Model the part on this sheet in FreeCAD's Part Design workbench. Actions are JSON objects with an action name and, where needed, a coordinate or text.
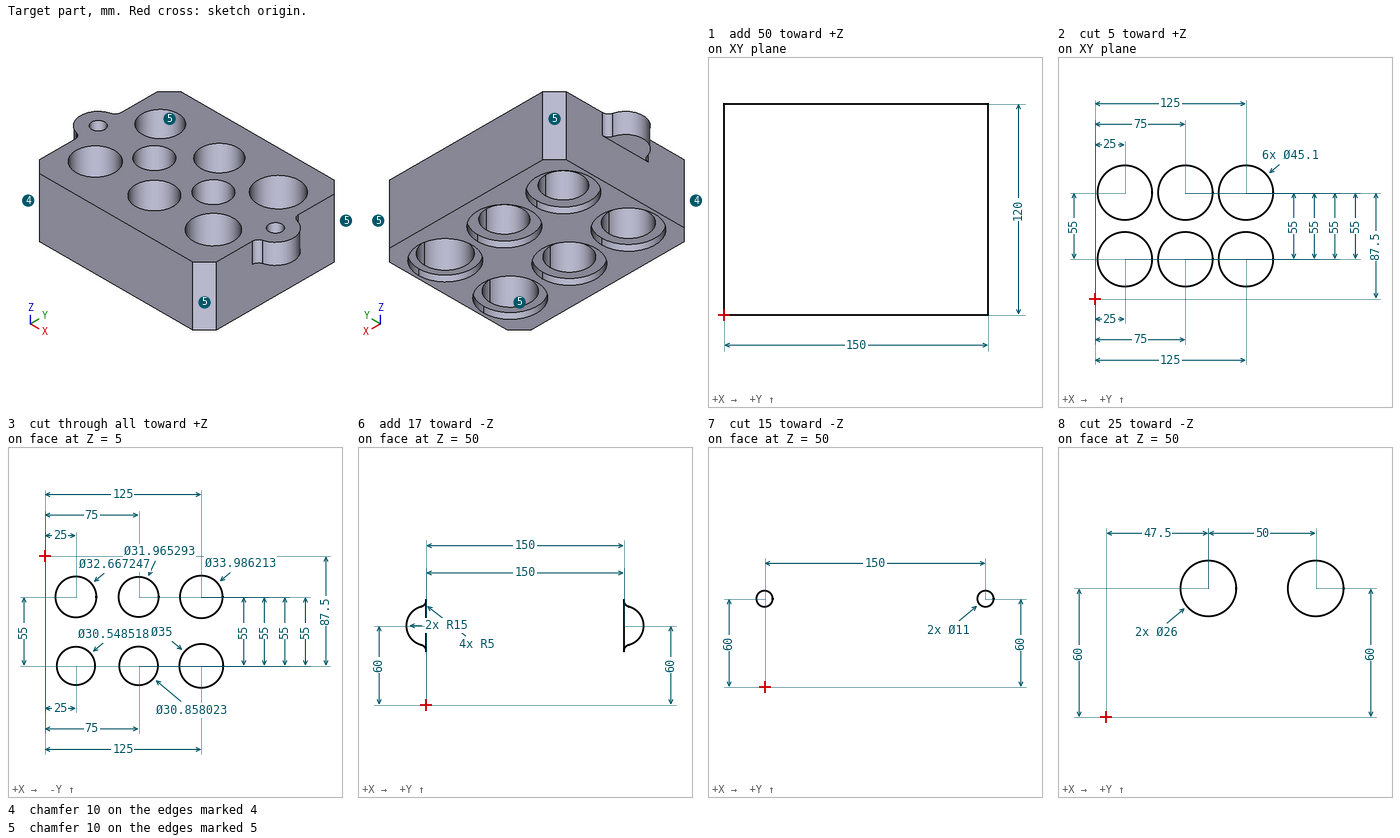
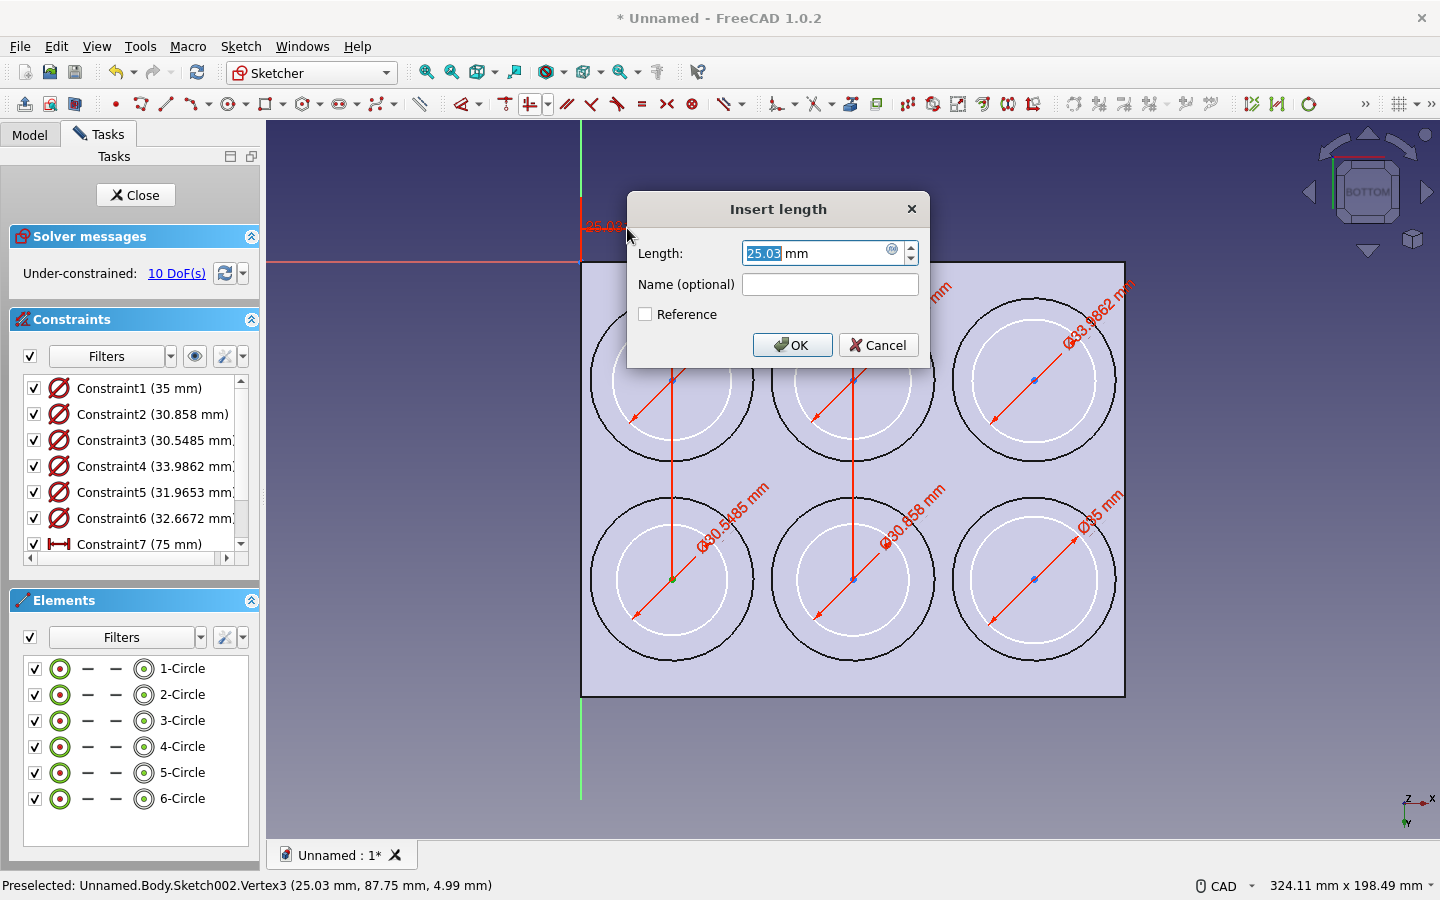
{"action": "type", "text": "25"}
{"action": "key", "text": "Return"}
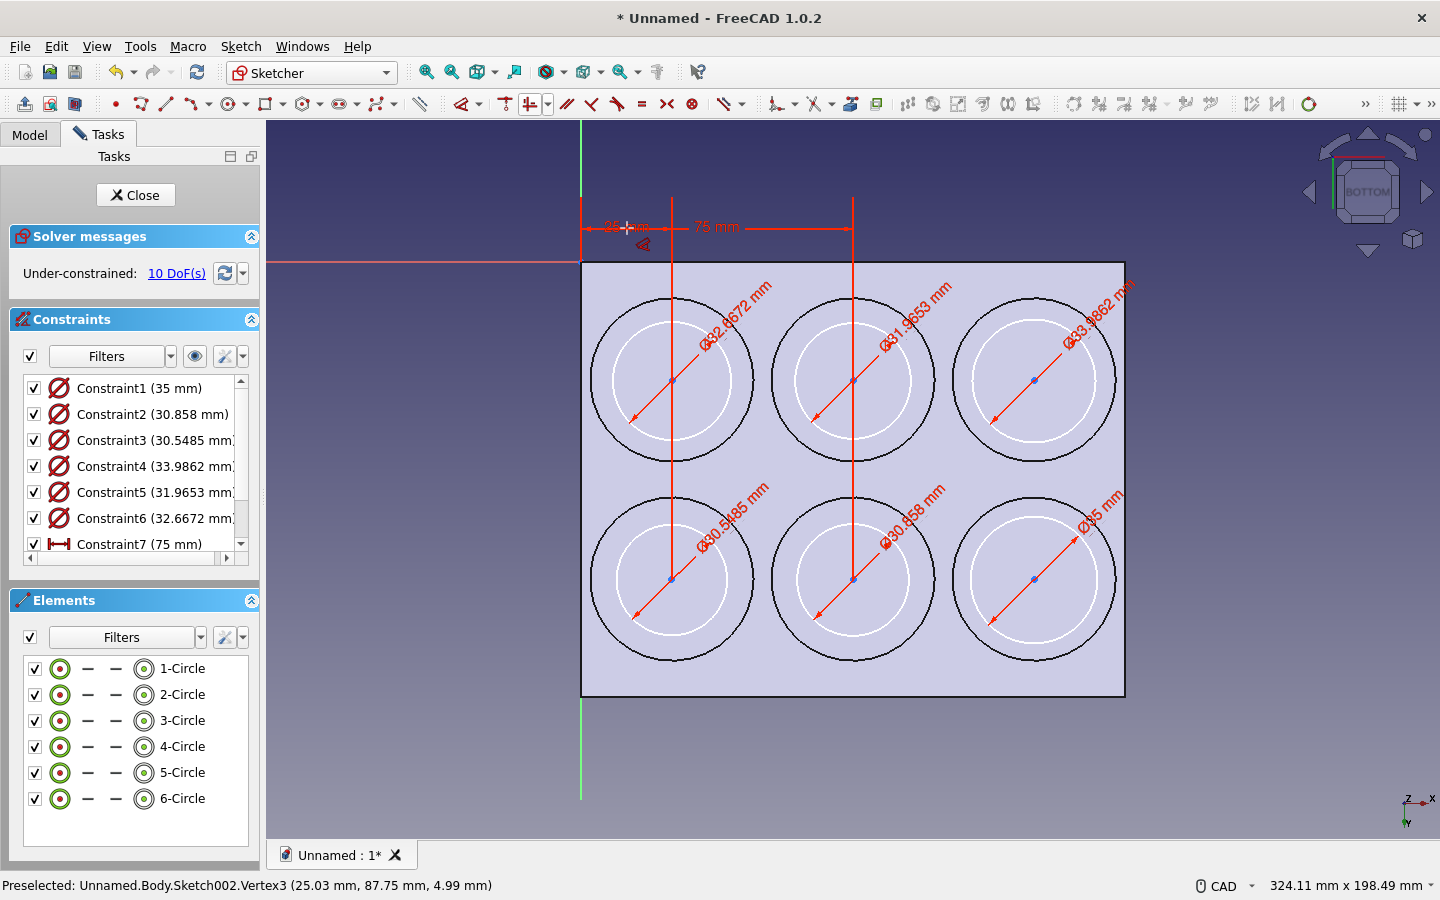
{"action": "left_click", "coordinate": [853, 381]}
{"action": "left_click", "coordinate": [812, 228]}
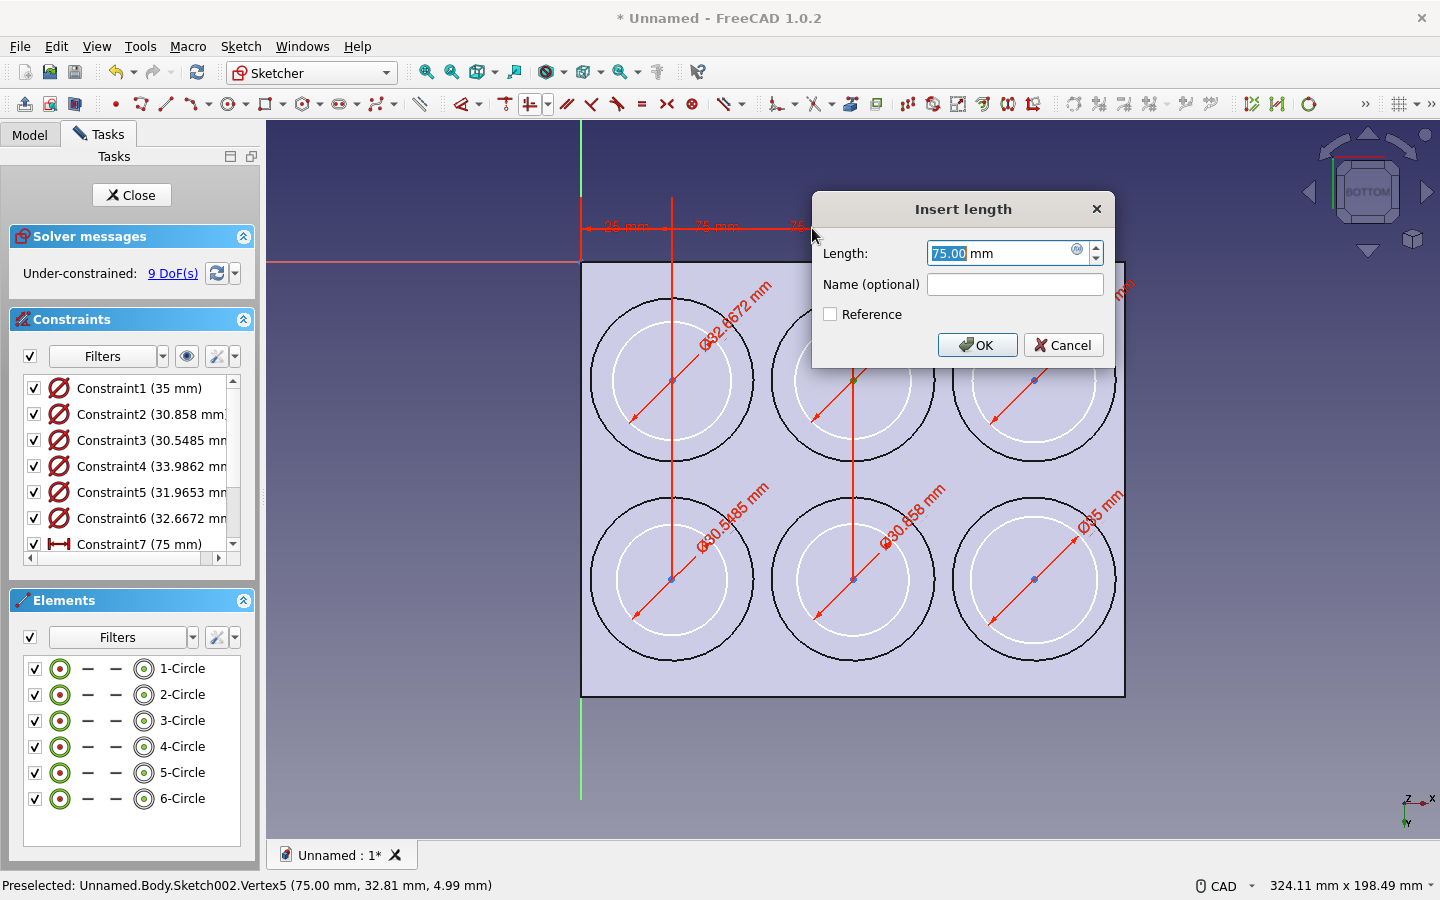
{"action": "type", "text": "75"}
{"action": "key", "text": "Return"}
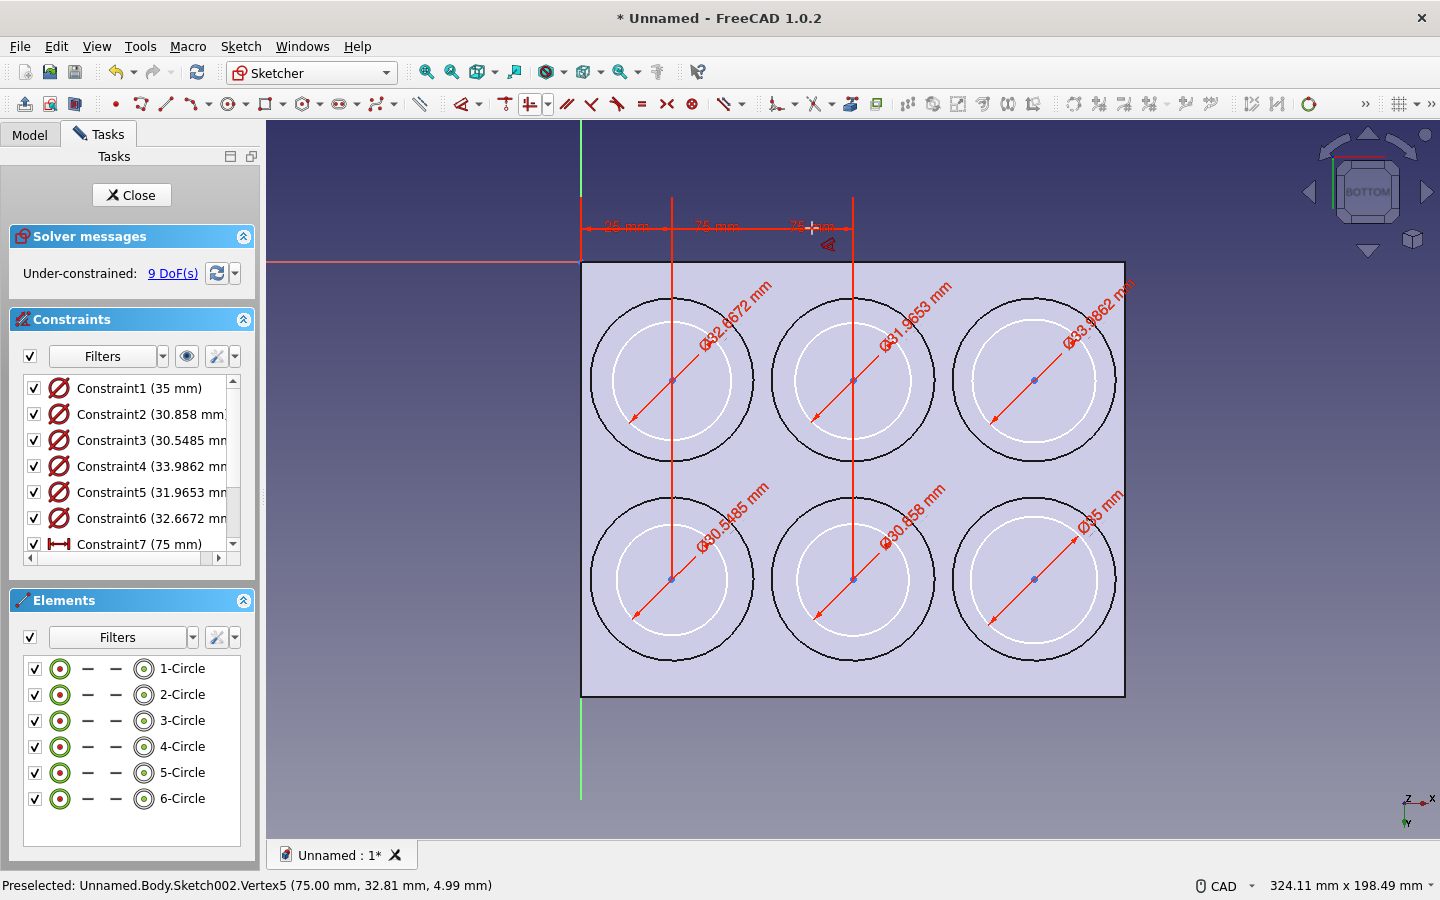
{"action": "left_click", "coordinate": [672, 381]}
{"action": "left_click", "coordinate": [606, 415]}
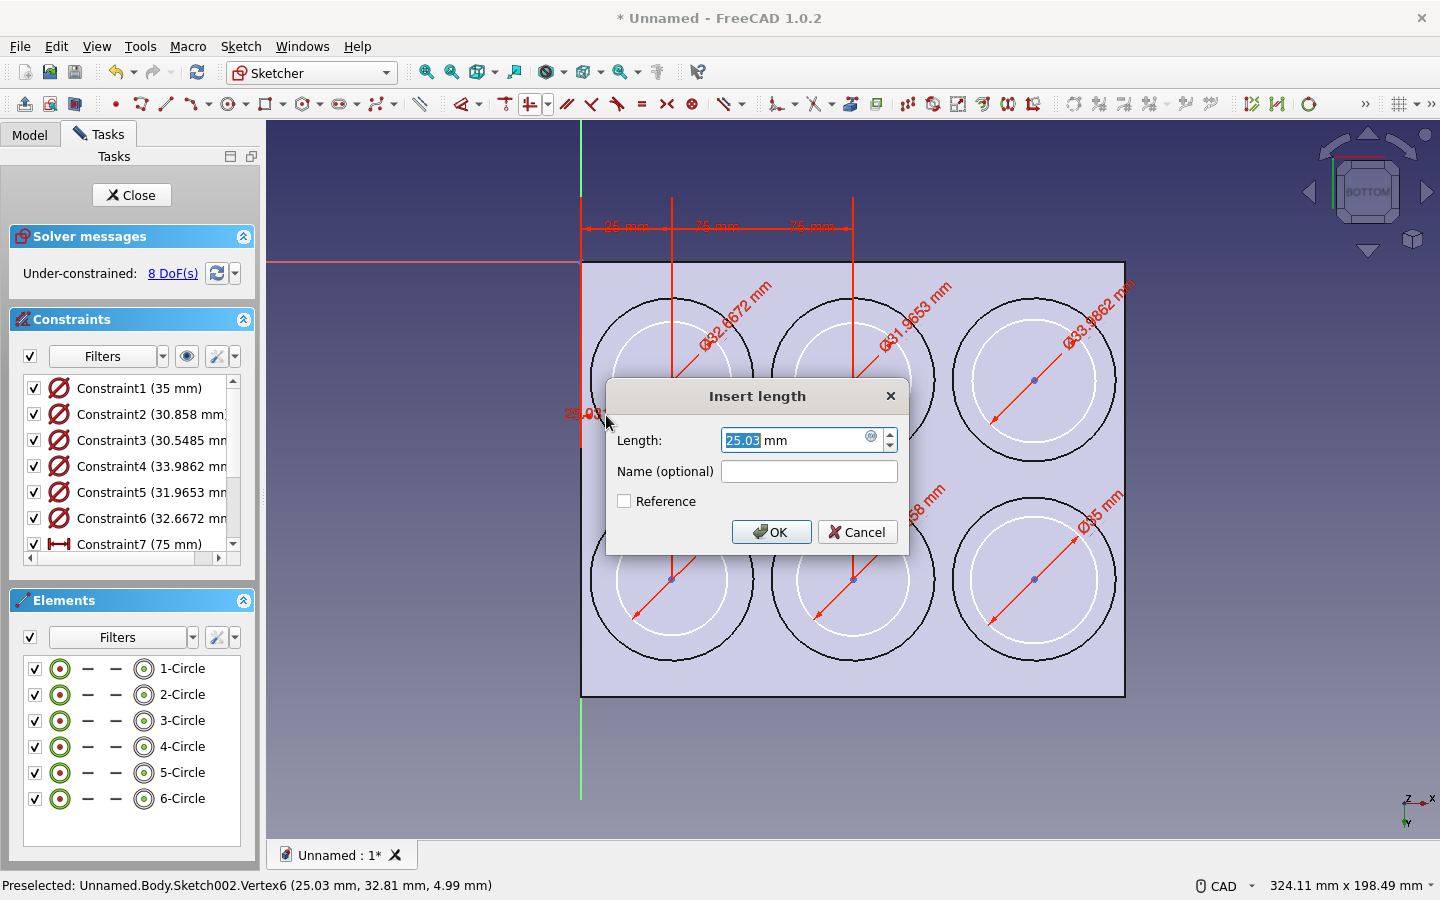
{"action": "type", "text": "25"}
{"action": "key", "text": "Return"}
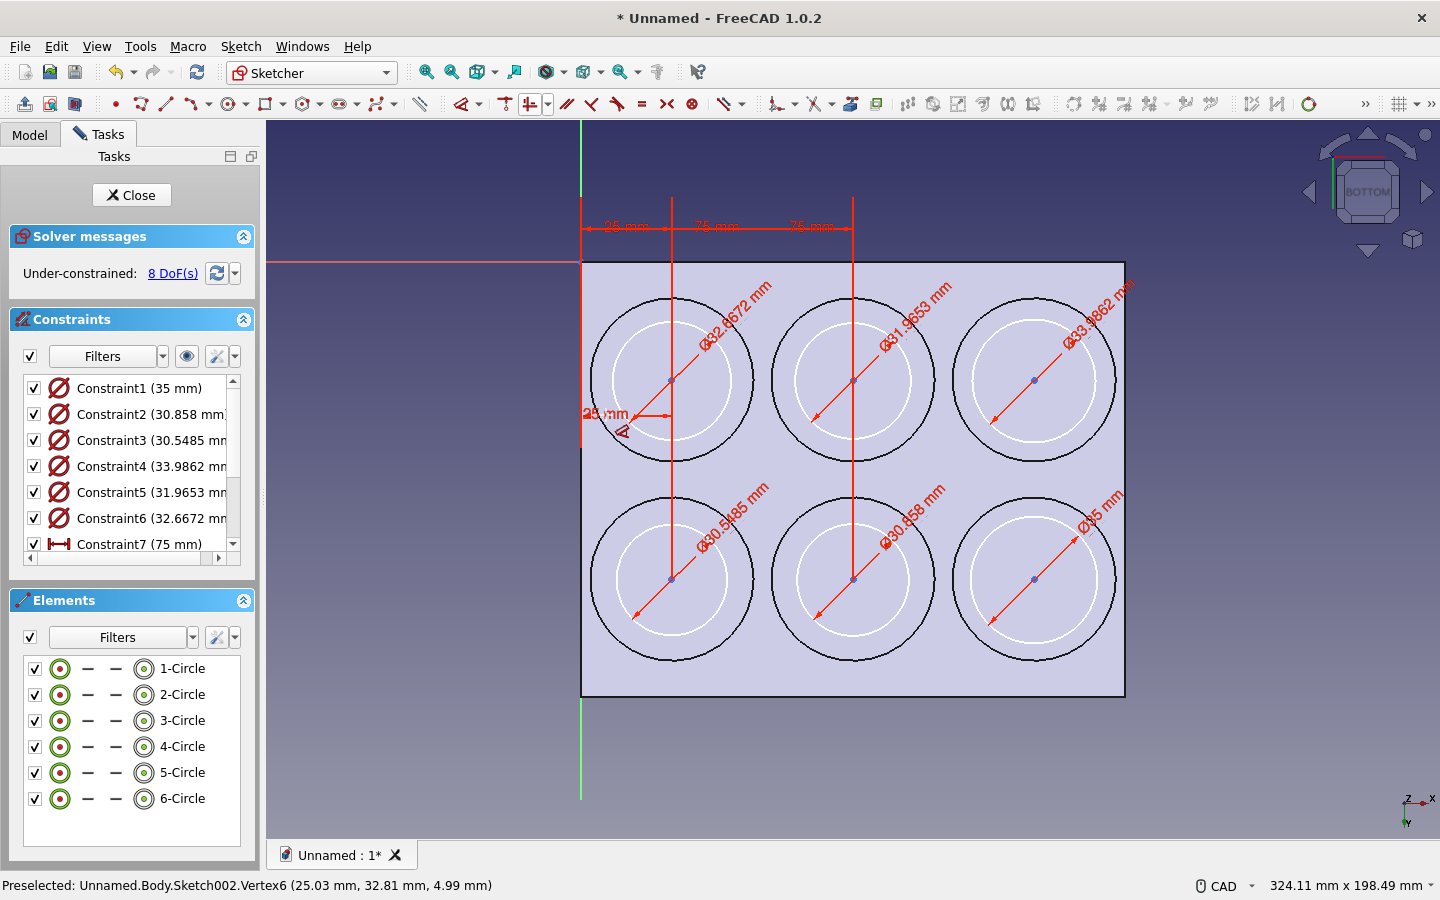
{"action": "left_click", "coordinate": [1034, 580]}
{"action": "left_click", "coordinate": [912, 228]}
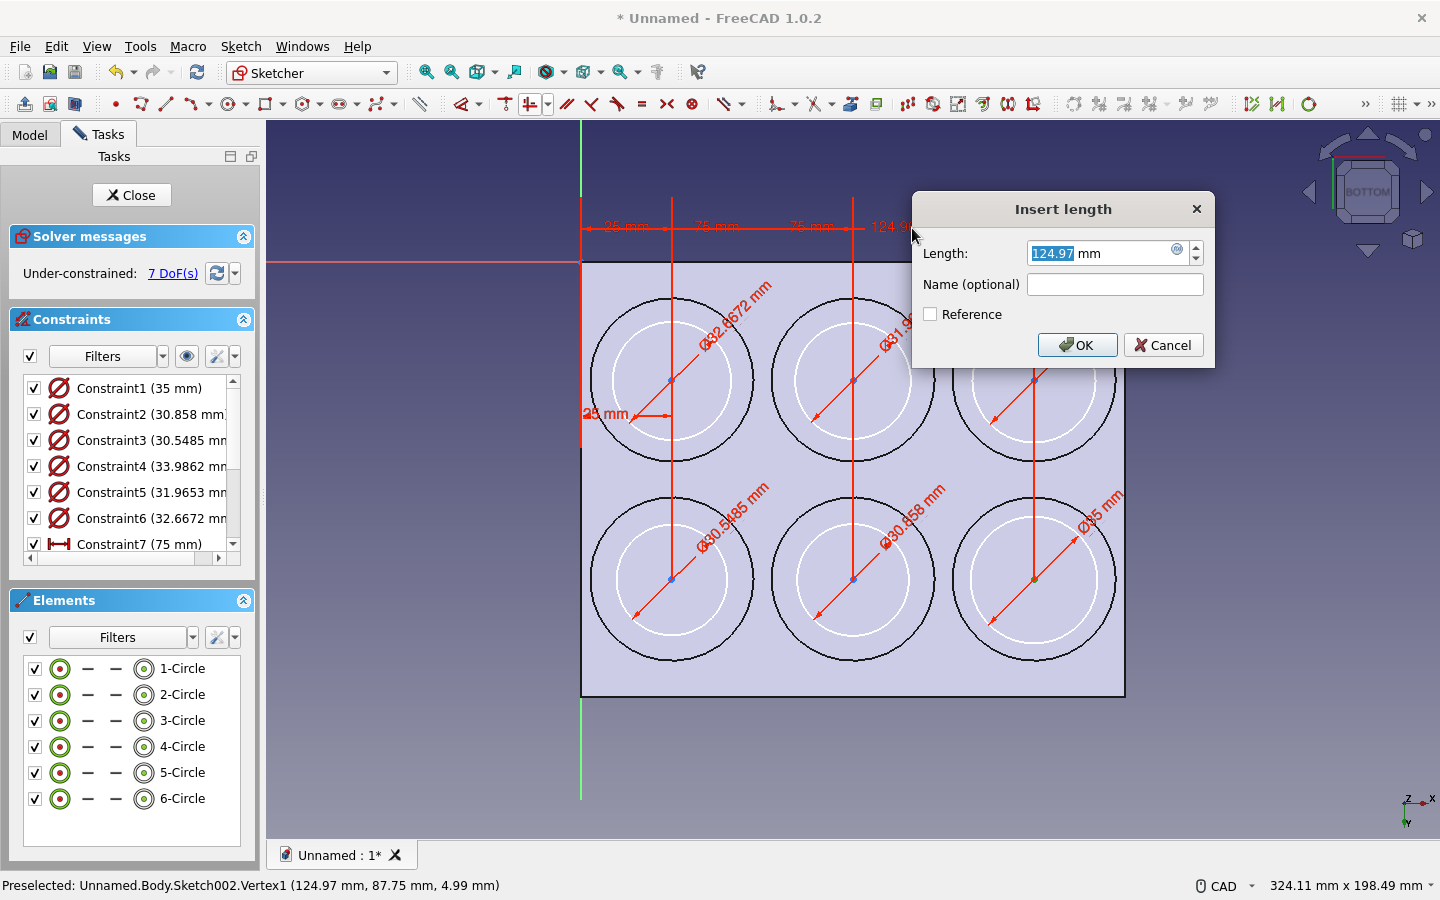
{"action": "type", "text": "125"}
{"action": "key", "text": "Return"}